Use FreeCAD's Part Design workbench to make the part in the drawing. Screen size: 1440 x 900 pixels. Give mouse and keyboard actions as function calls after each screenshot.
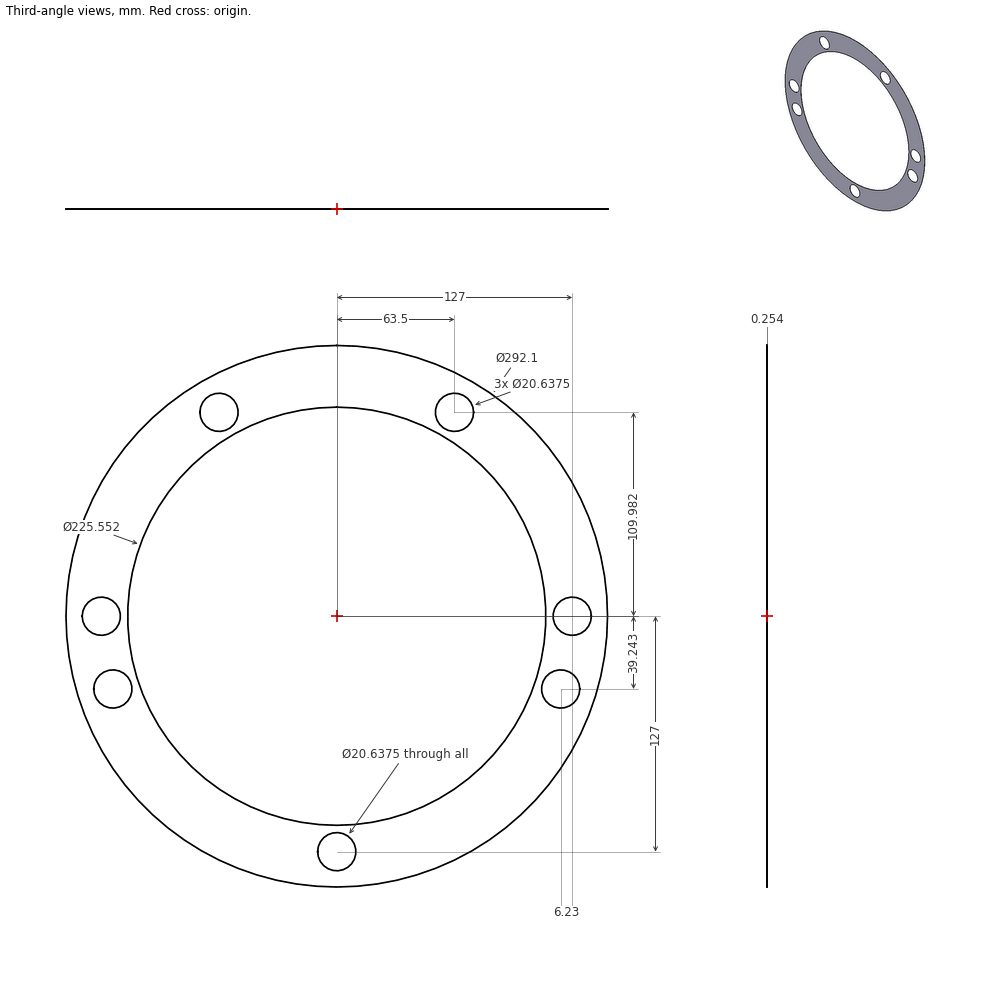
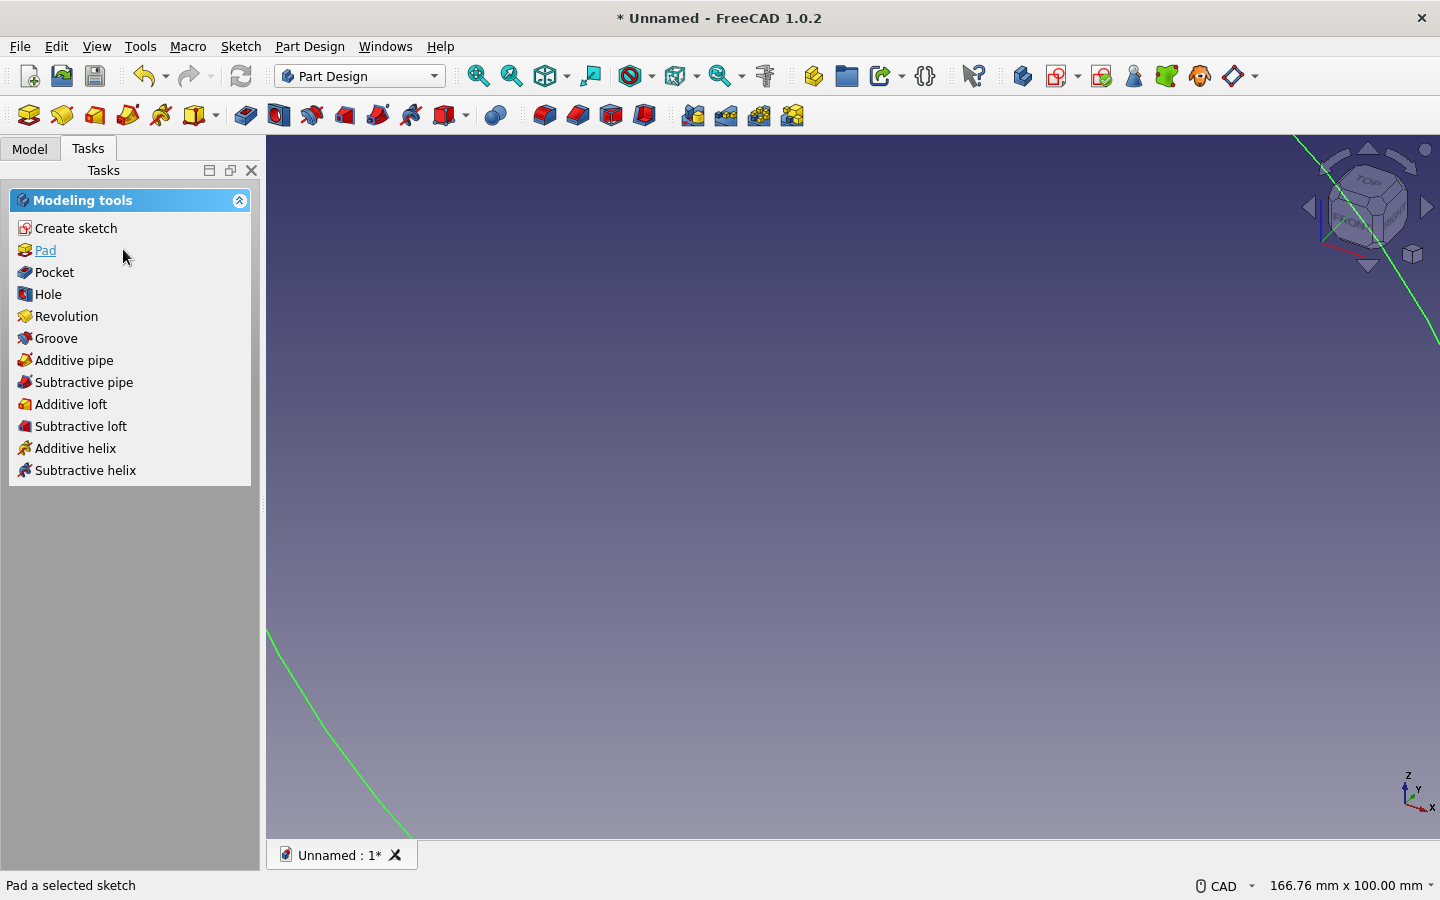
click(29, 116)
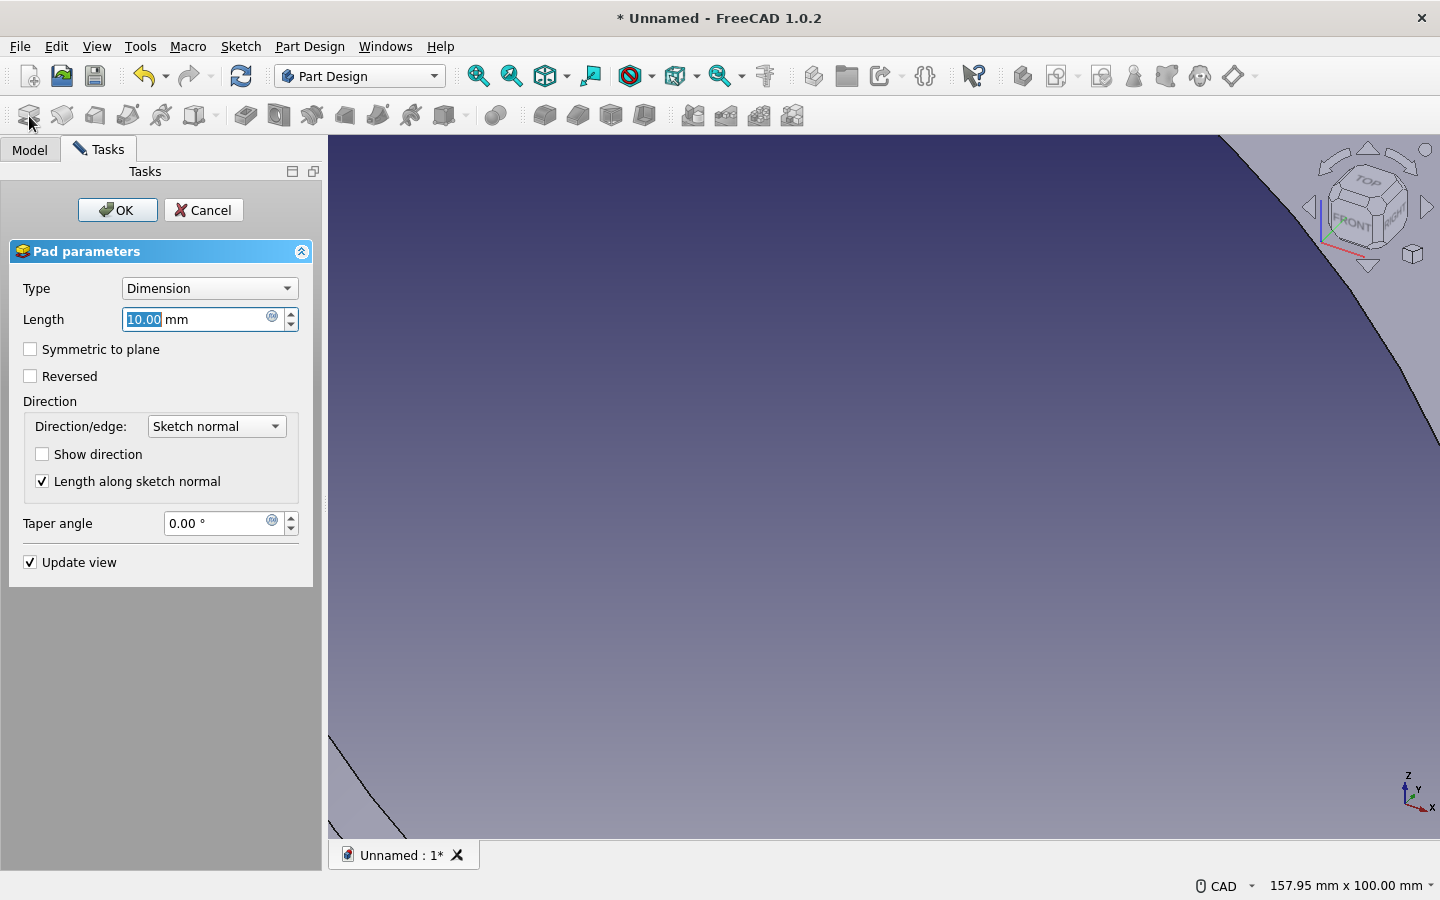
text(0.254)
key(Tab)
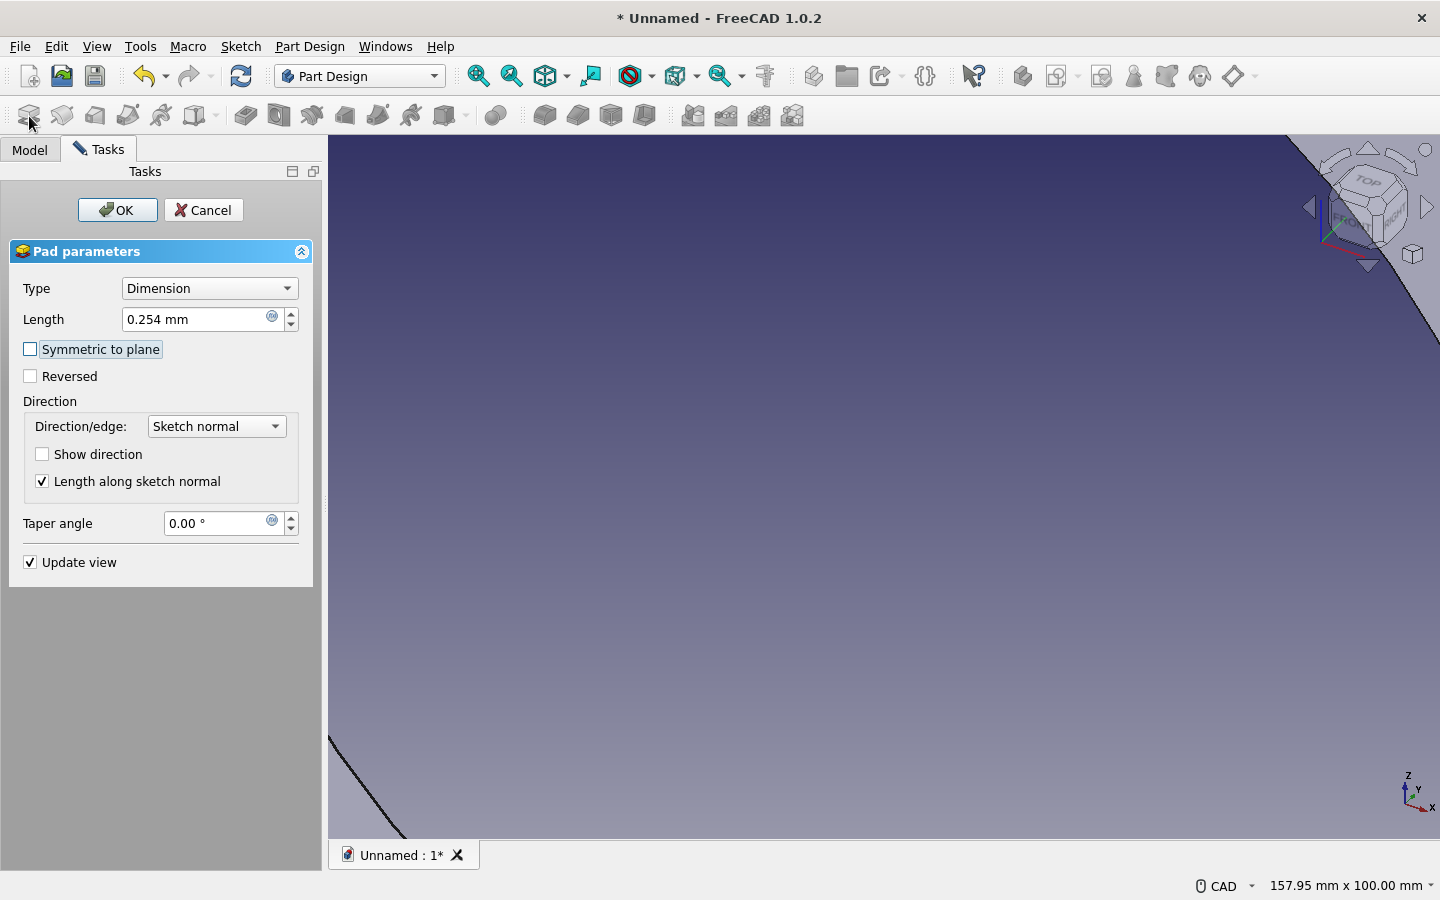
click(31, 376)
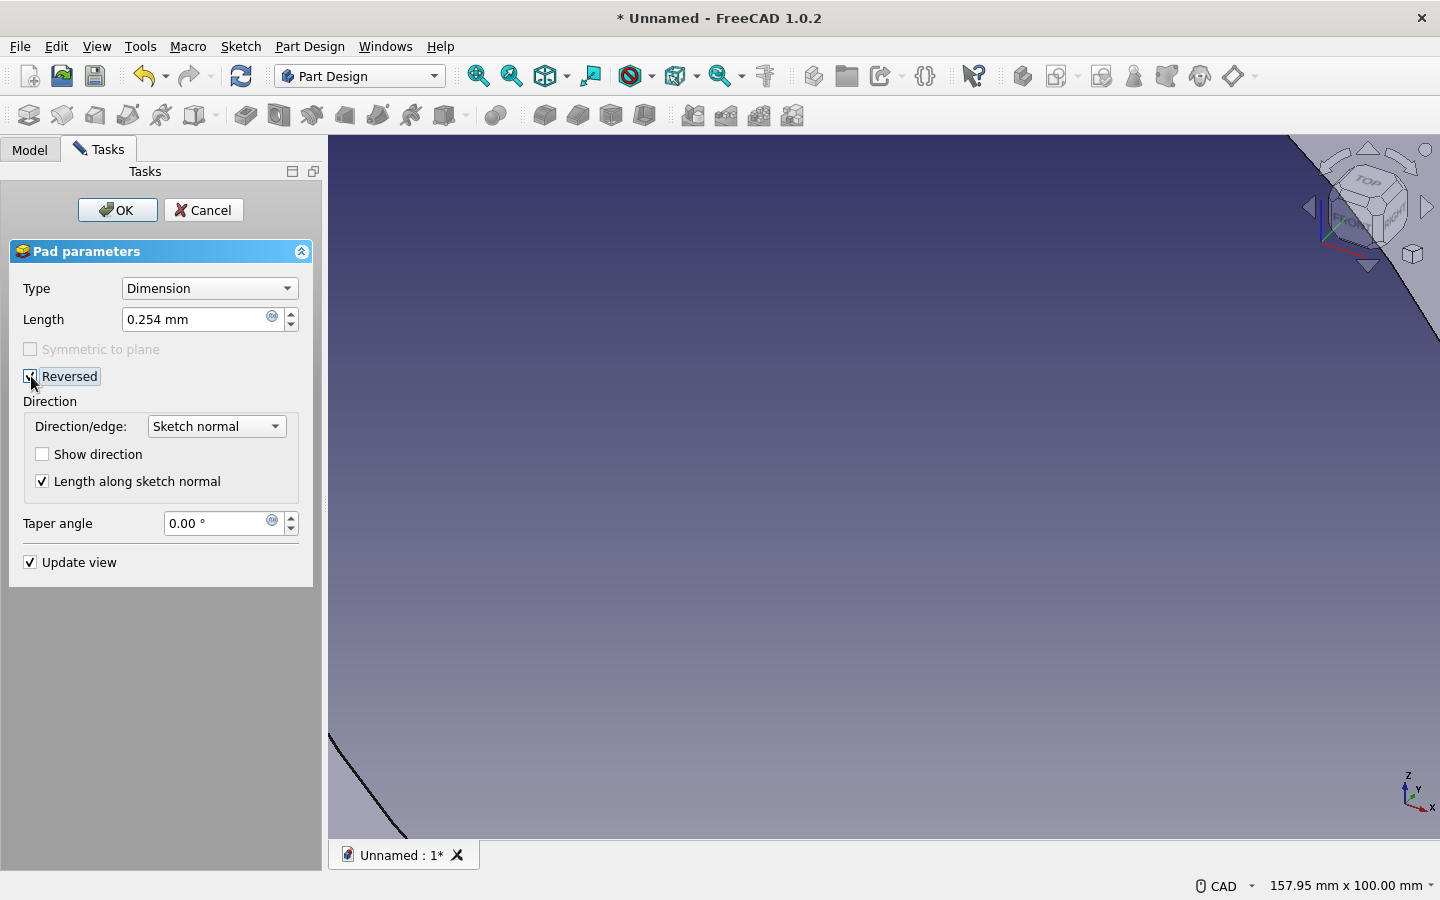
click(118, 210)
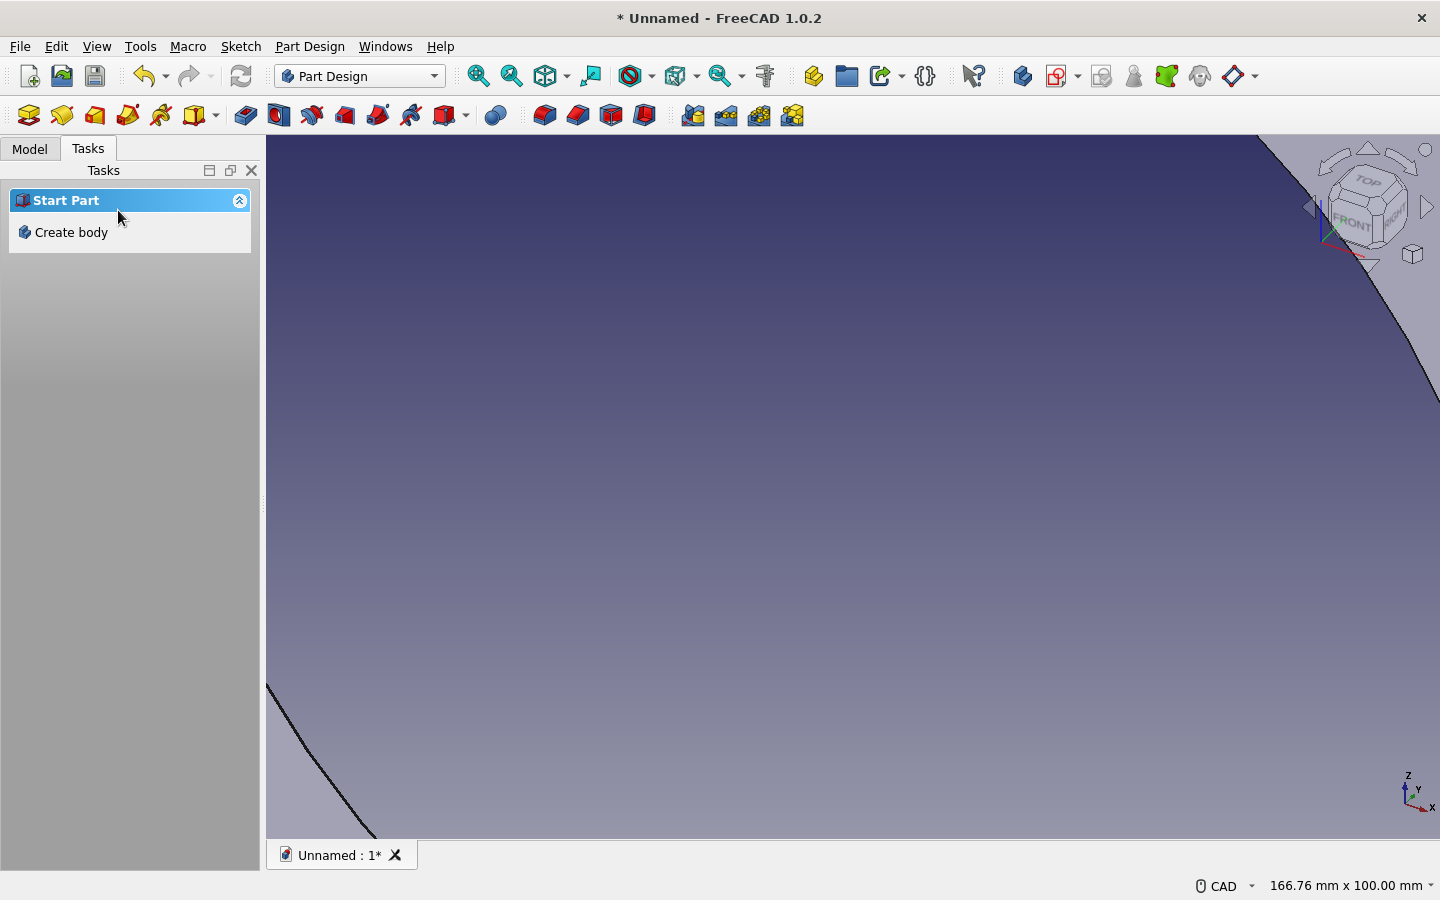
click(479, 76)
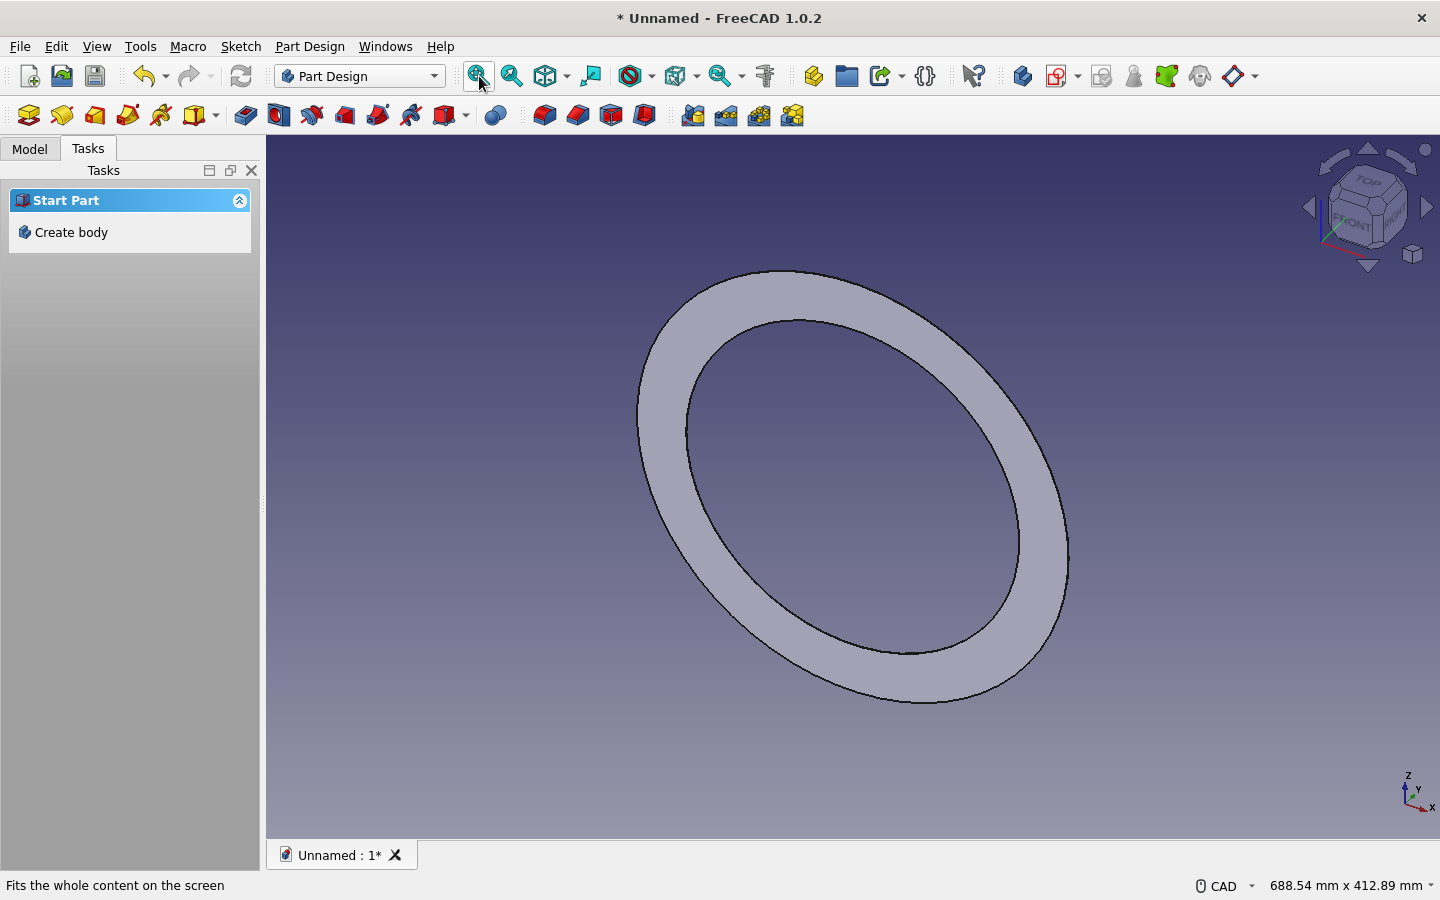
key(4)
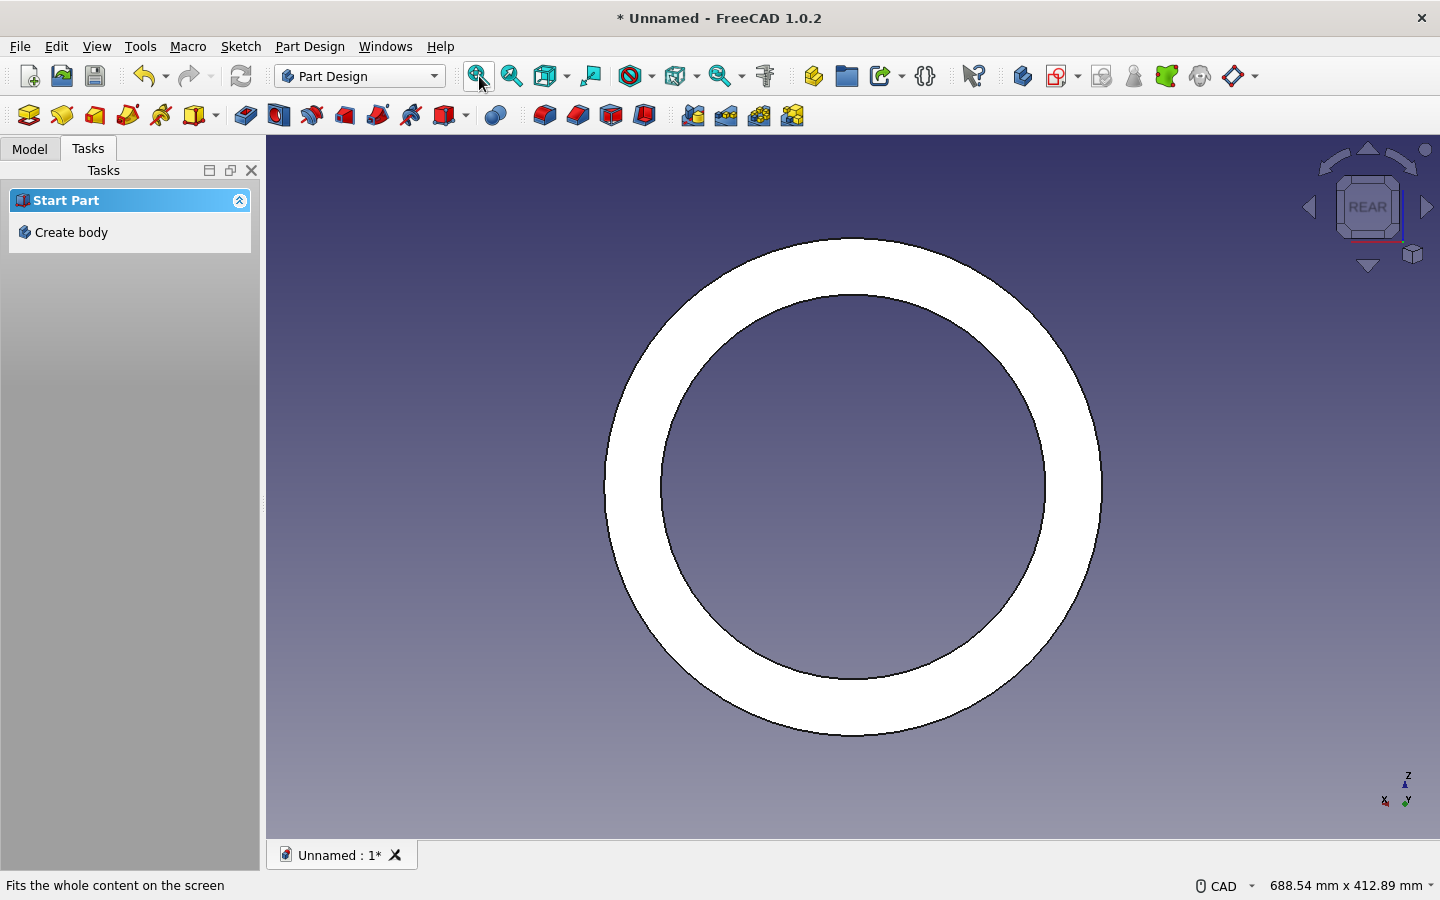
click(782, 699)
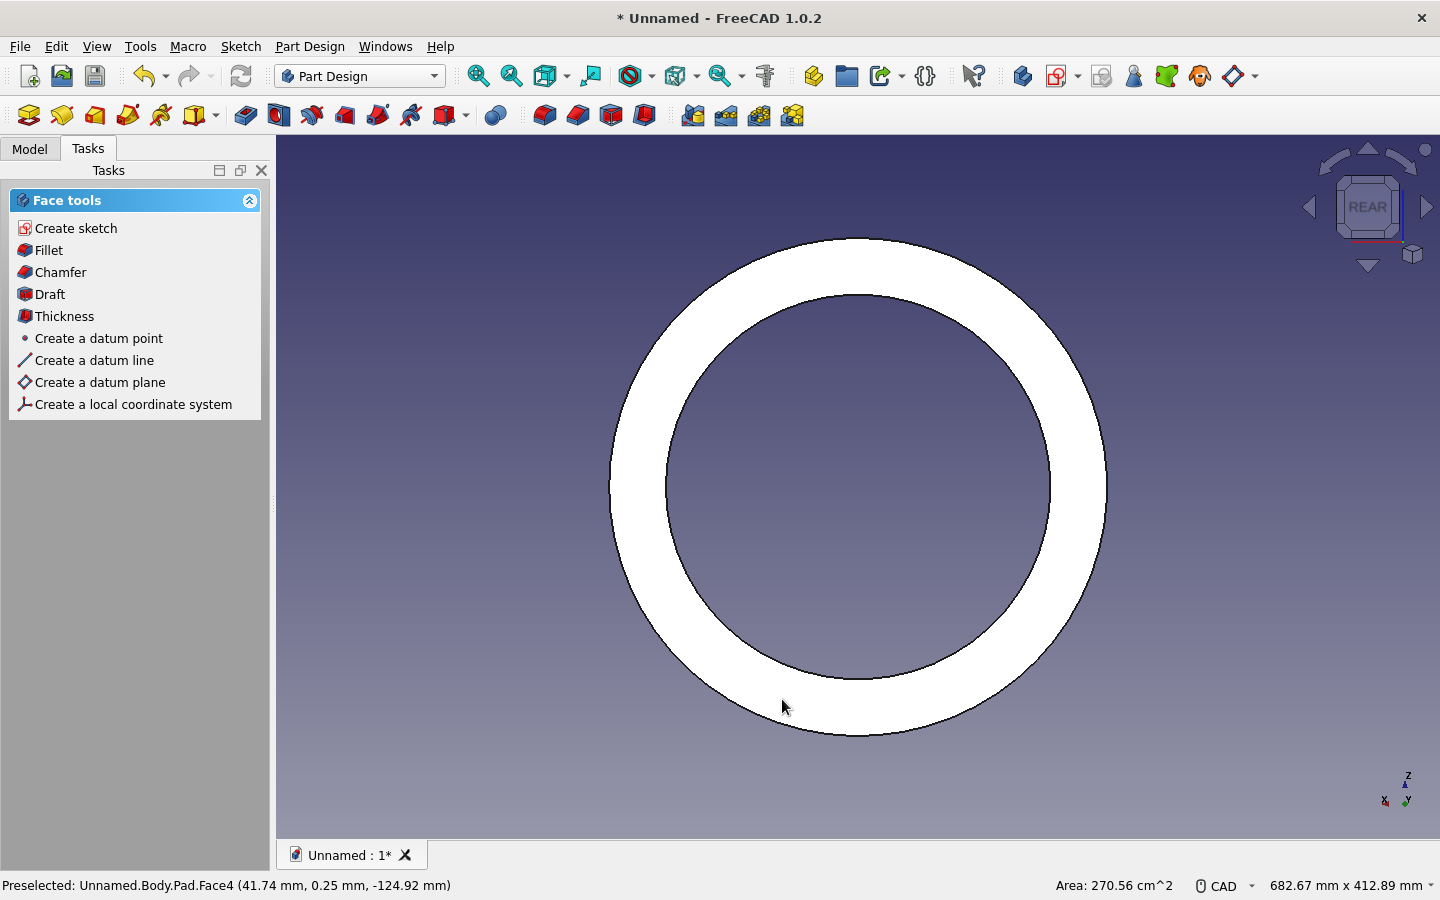
click(1056, 76)